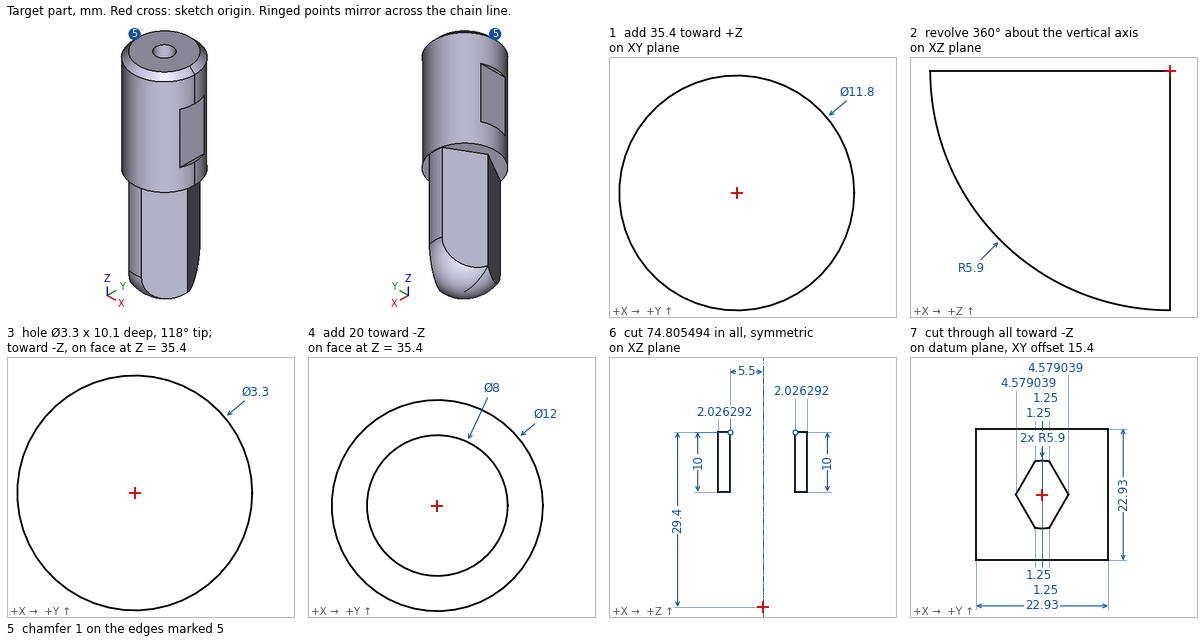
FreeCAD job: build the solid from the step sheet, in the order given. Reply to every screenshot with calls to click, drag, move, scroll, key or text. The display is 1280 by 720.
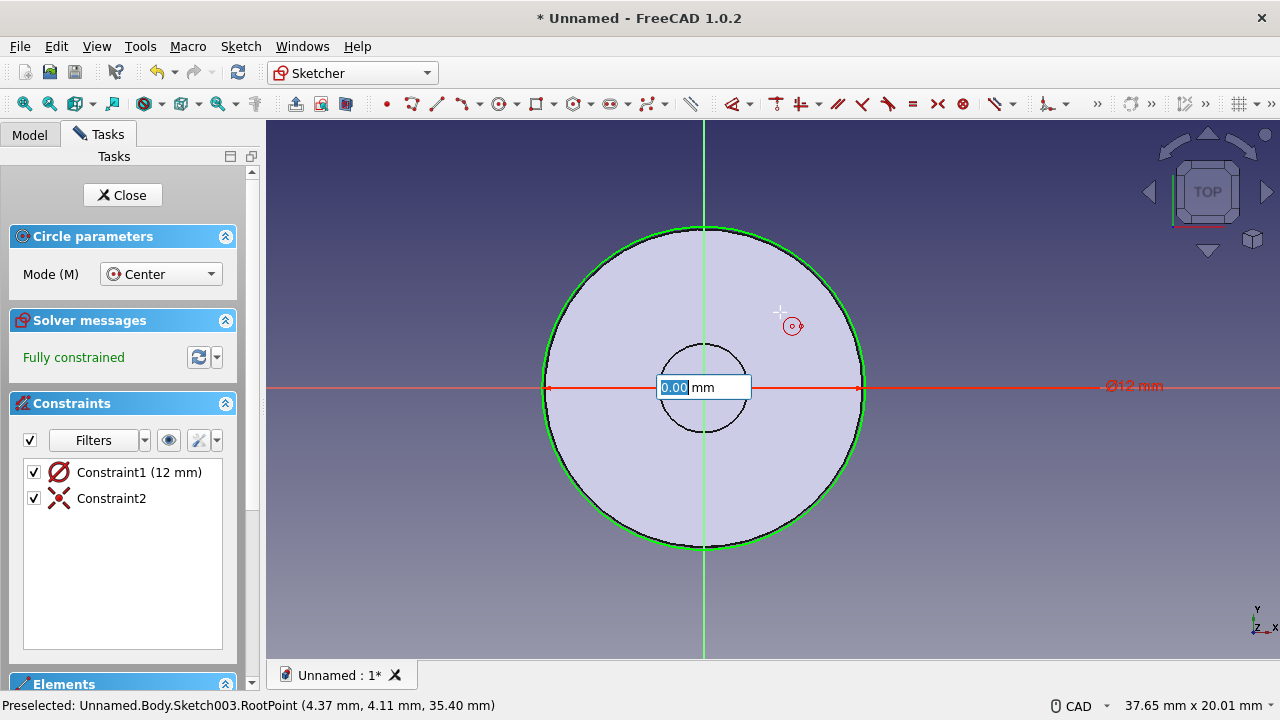
text(8)
key(Return)
key(Escape)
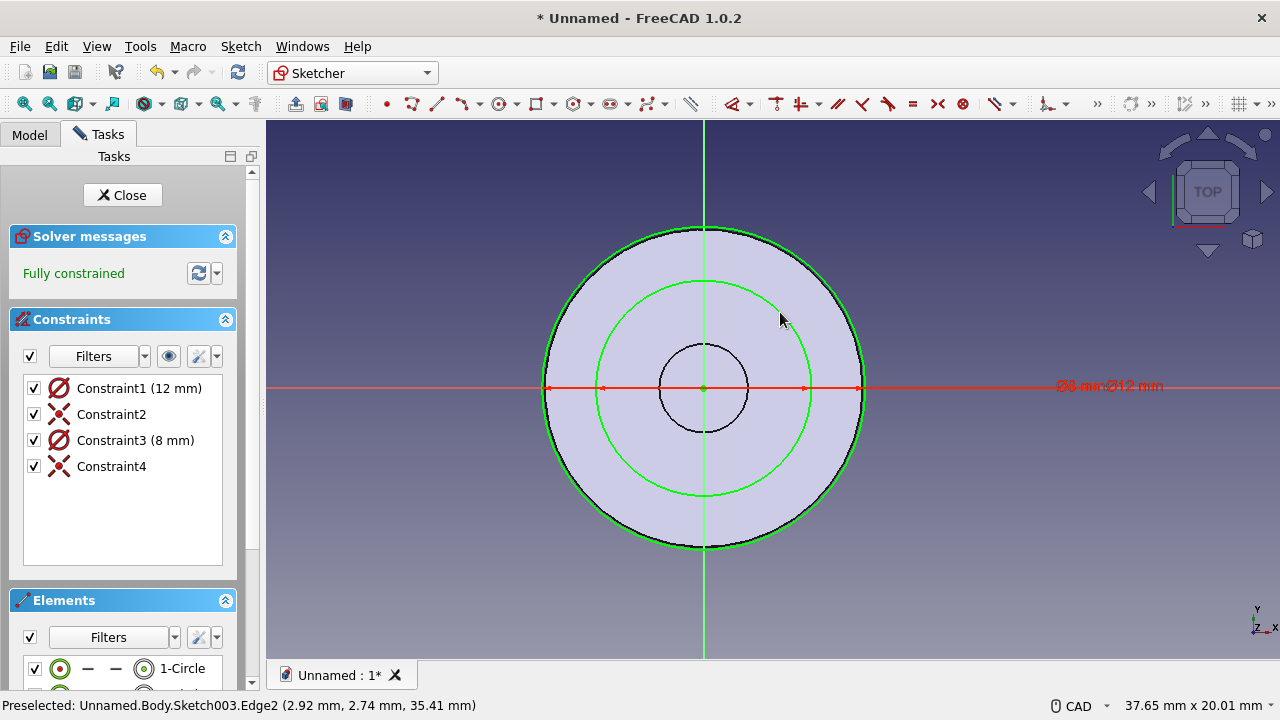
click(123, 195)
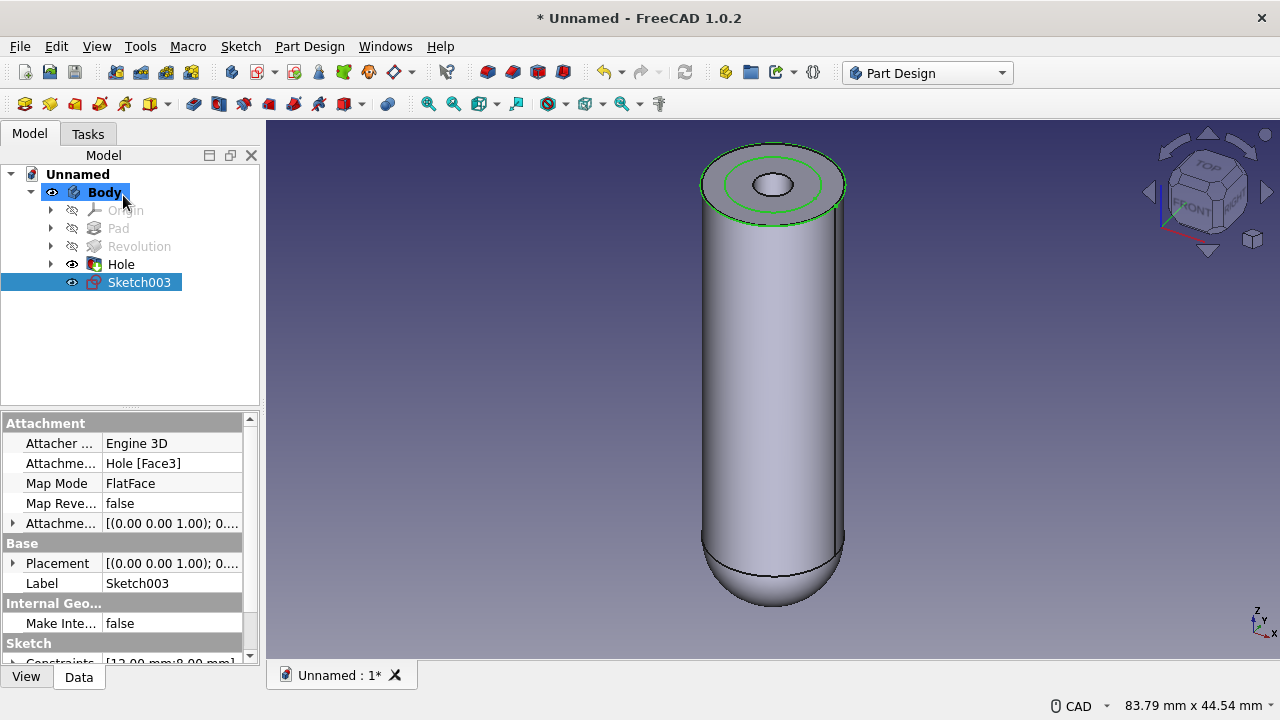
click(25, 104)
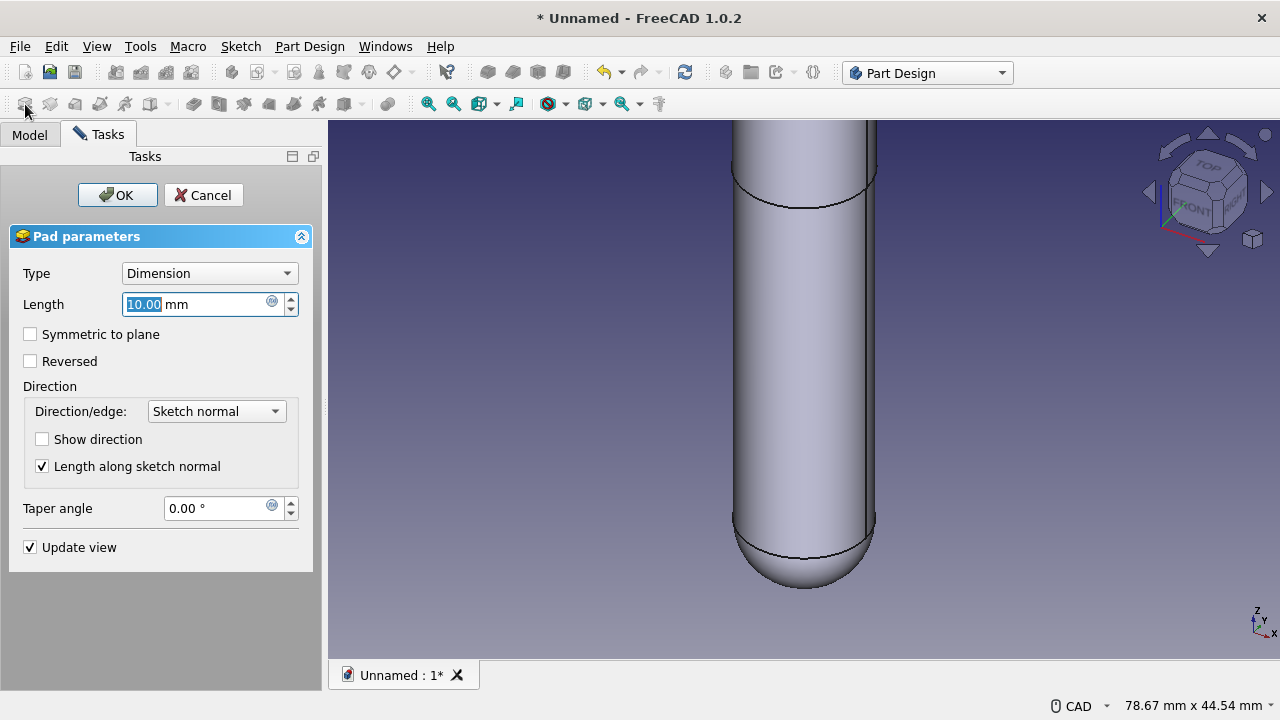
text(20)
key(Tab)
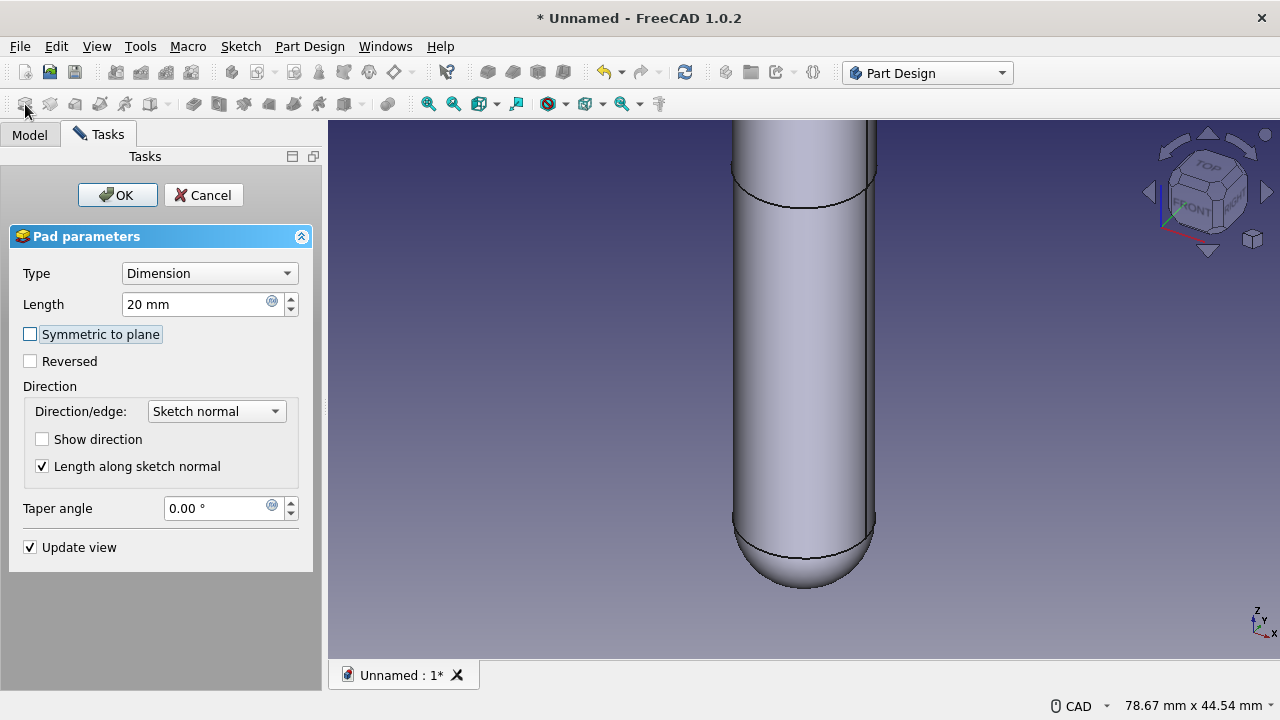
click(31, 361)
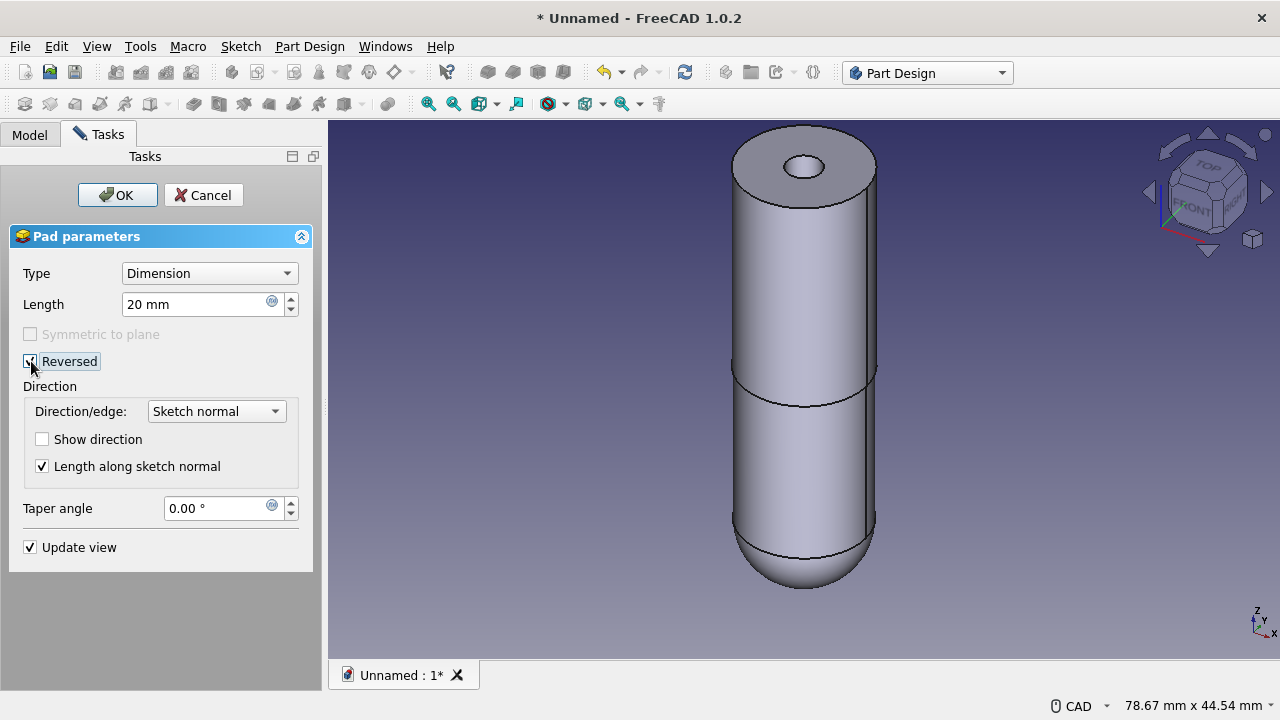
click(118, 195)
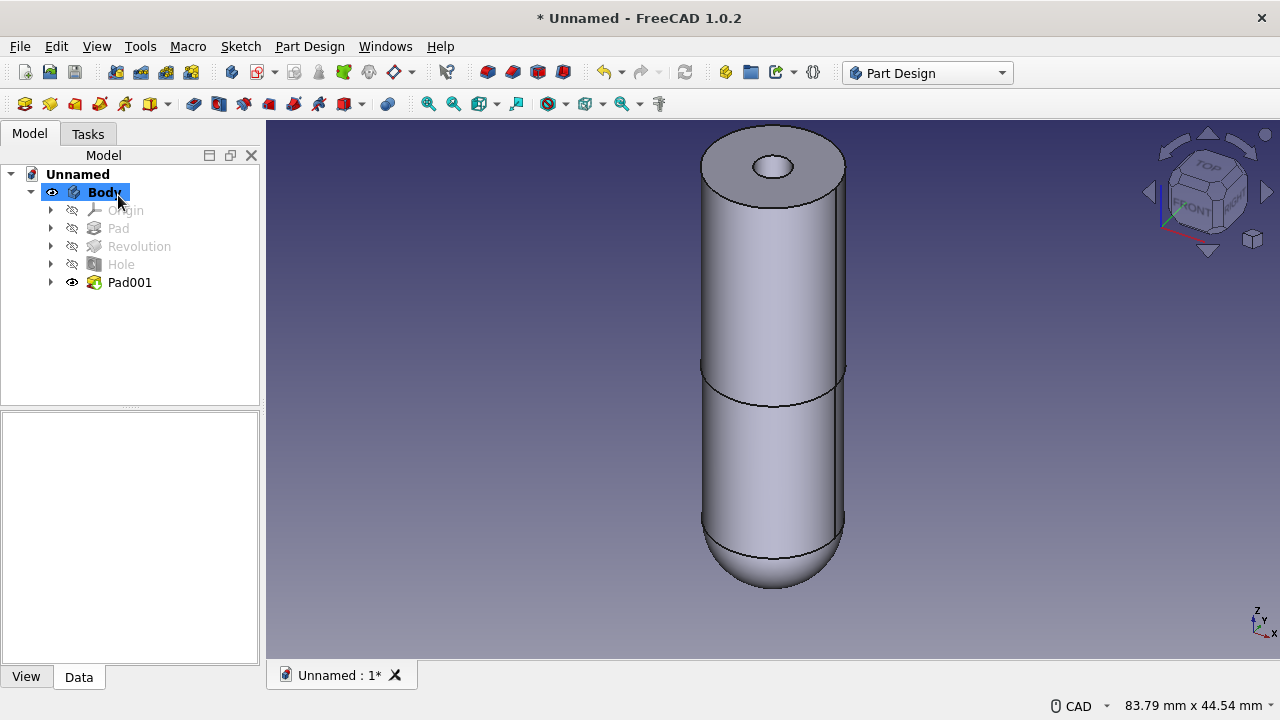
key(v)
key(f)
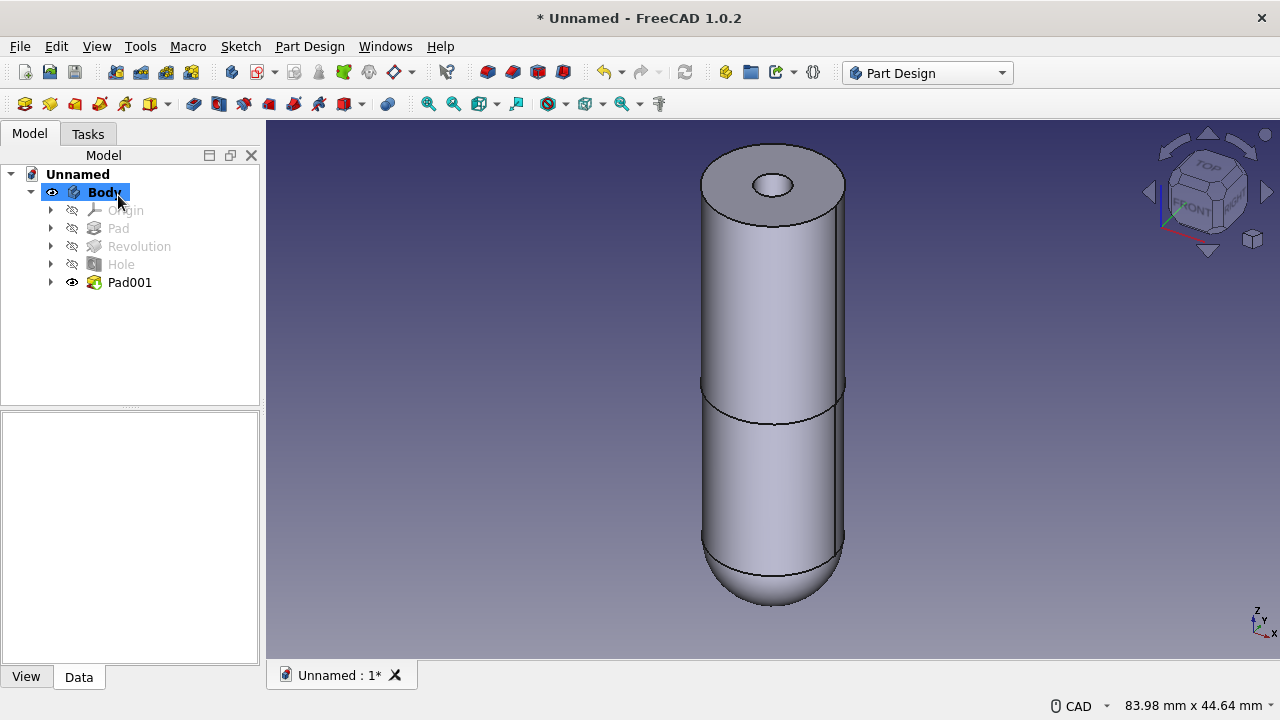
click(701, 189)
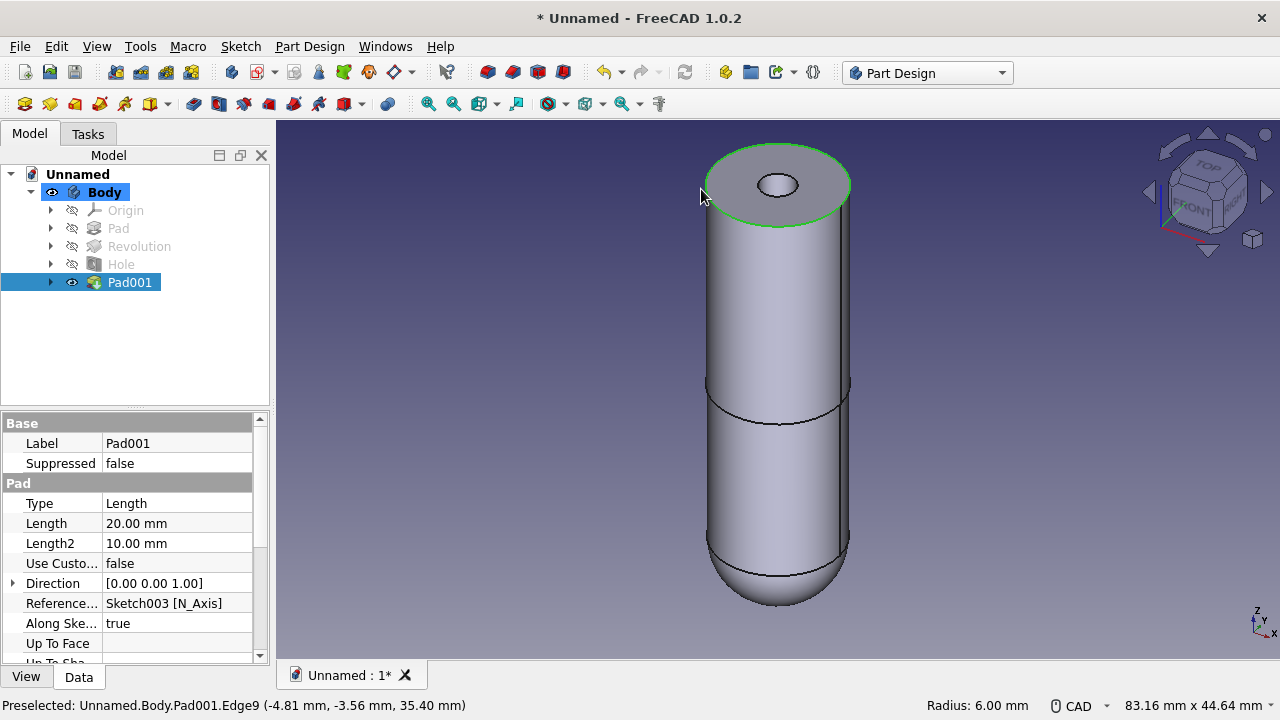
click(513, 72)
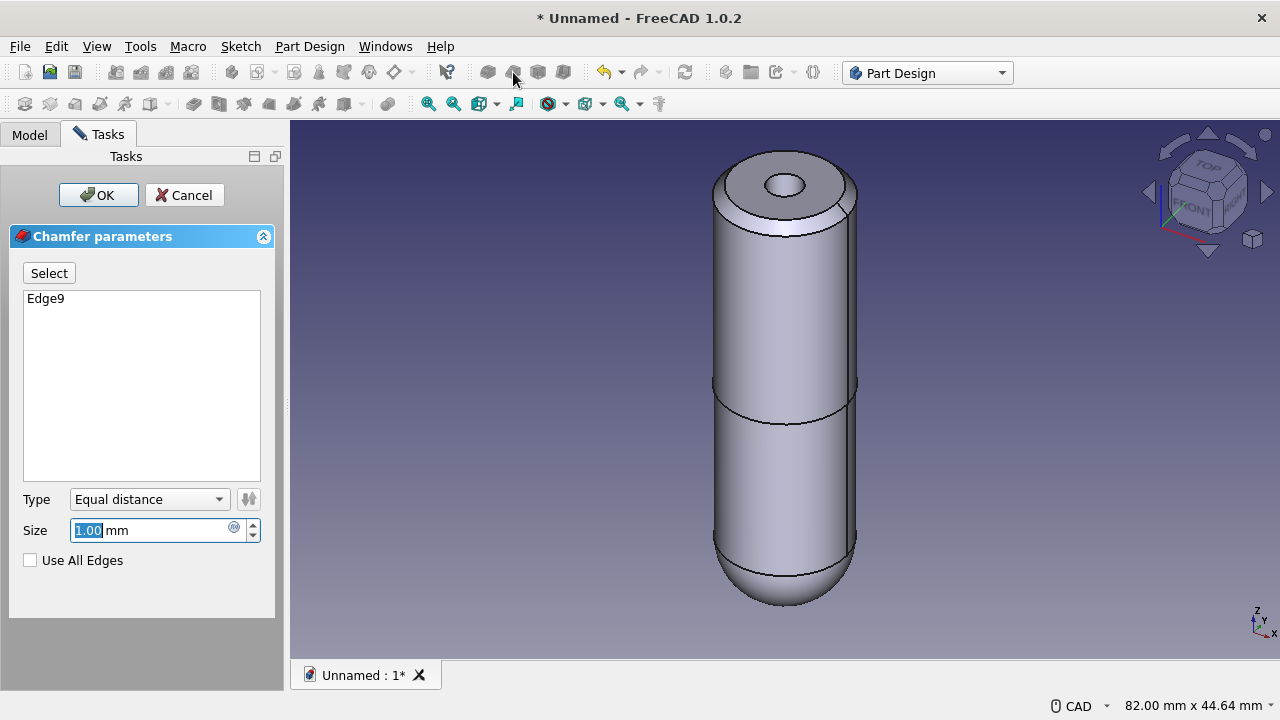
text(1)
key(Tab)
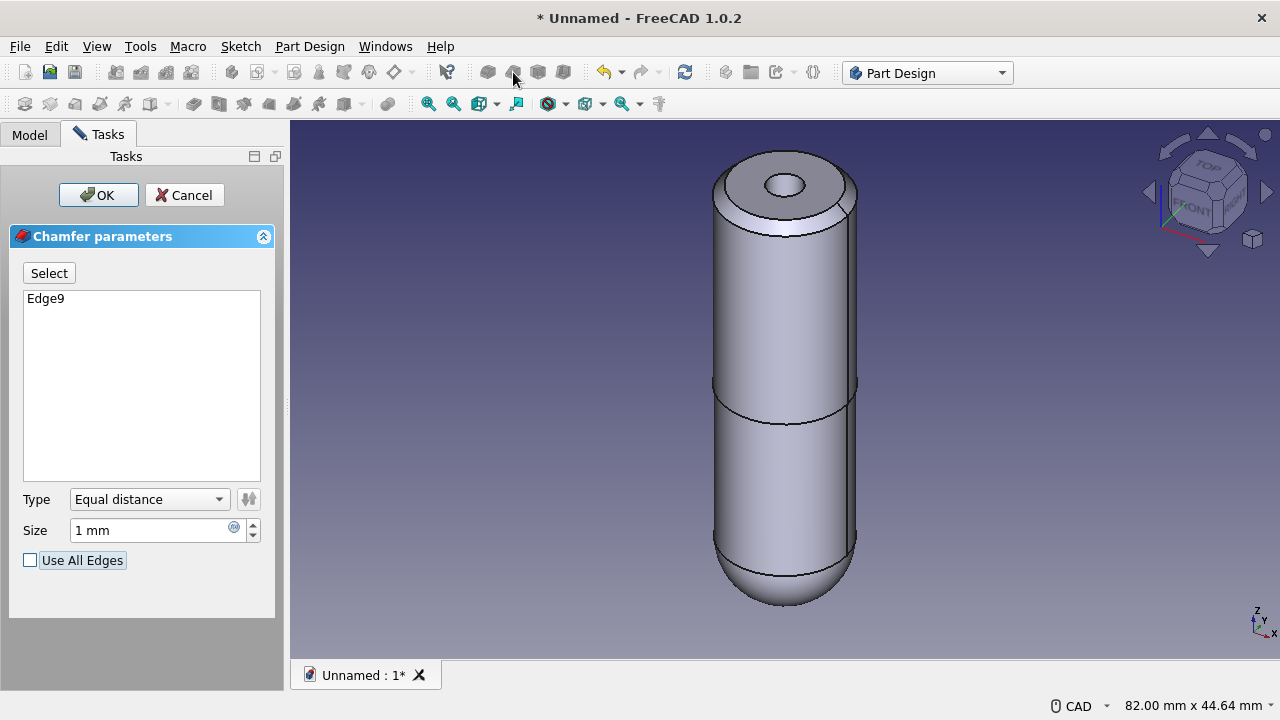
click(99, 195)